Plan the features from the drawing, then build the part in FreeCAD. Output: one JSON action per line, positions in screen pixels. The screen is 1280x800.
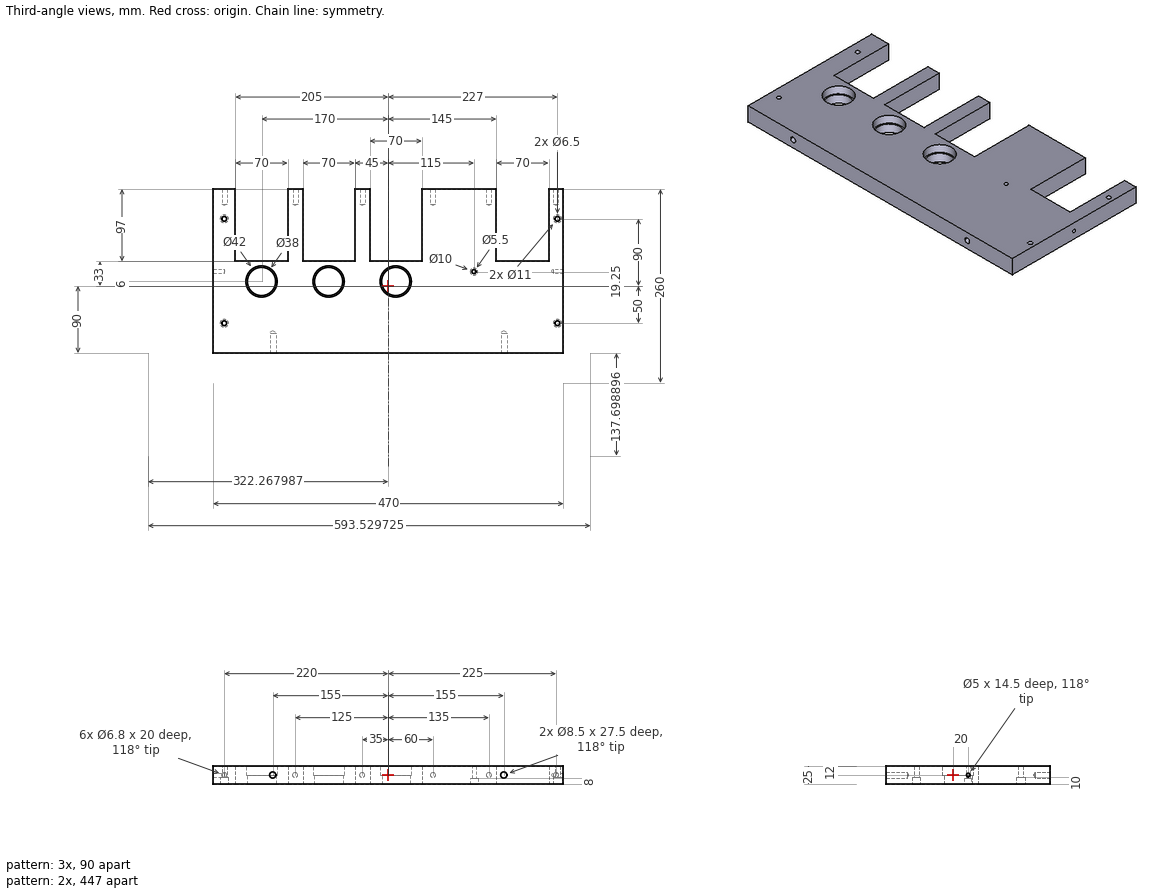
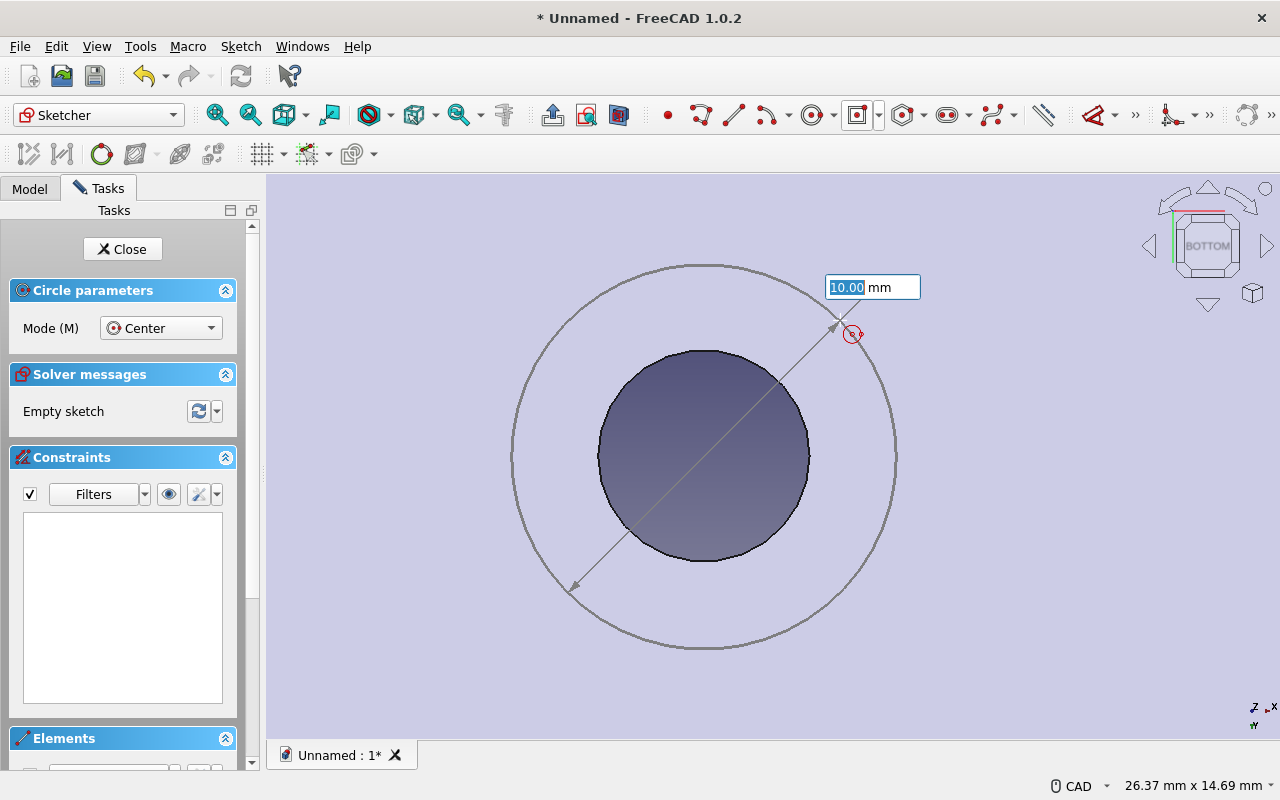
{"action": "type", "text": "10"}
{"action": "key", "text": "Return"}
{"action": "key", "text": "Escape"}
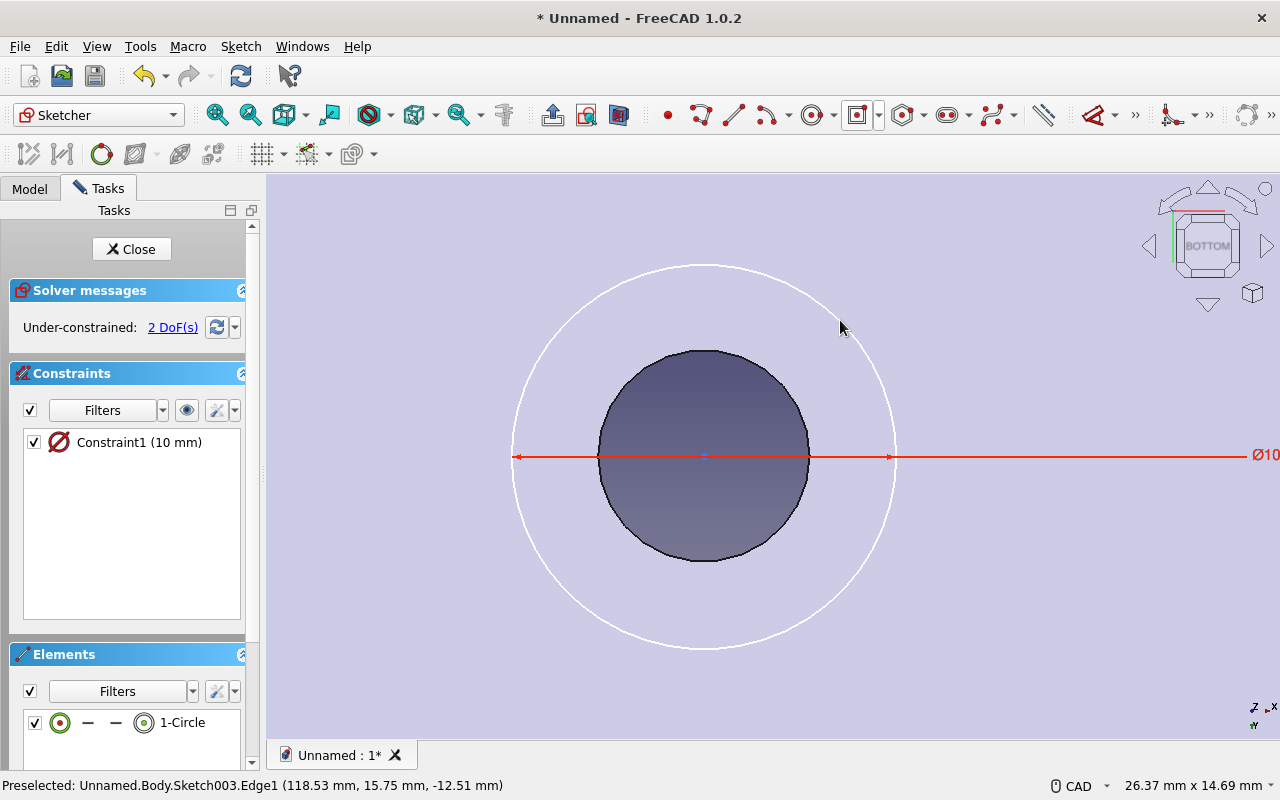
{"action": "left_click", "coordinate": [1092, 116]}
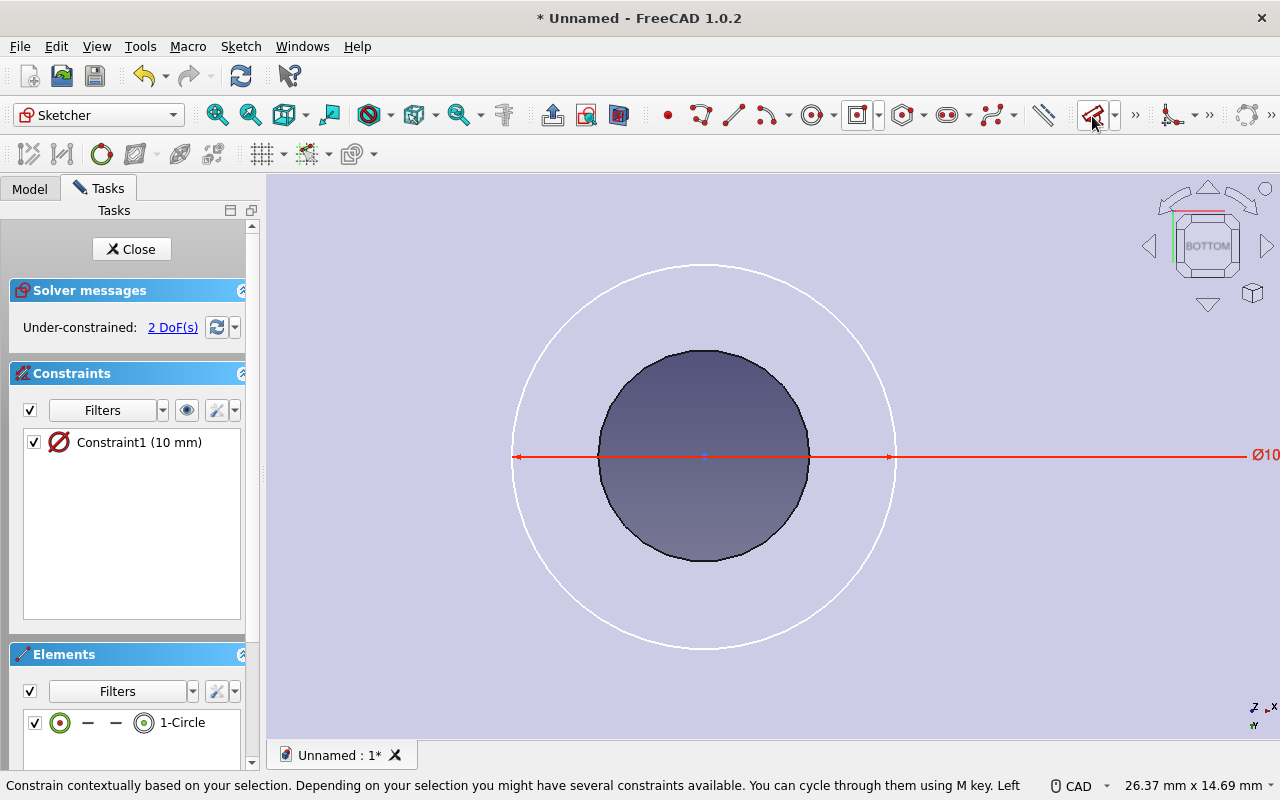
{"action": "left_click", "coordinate": [704, 457]}
{"action": "left_click", "coordinate": [499, 491]}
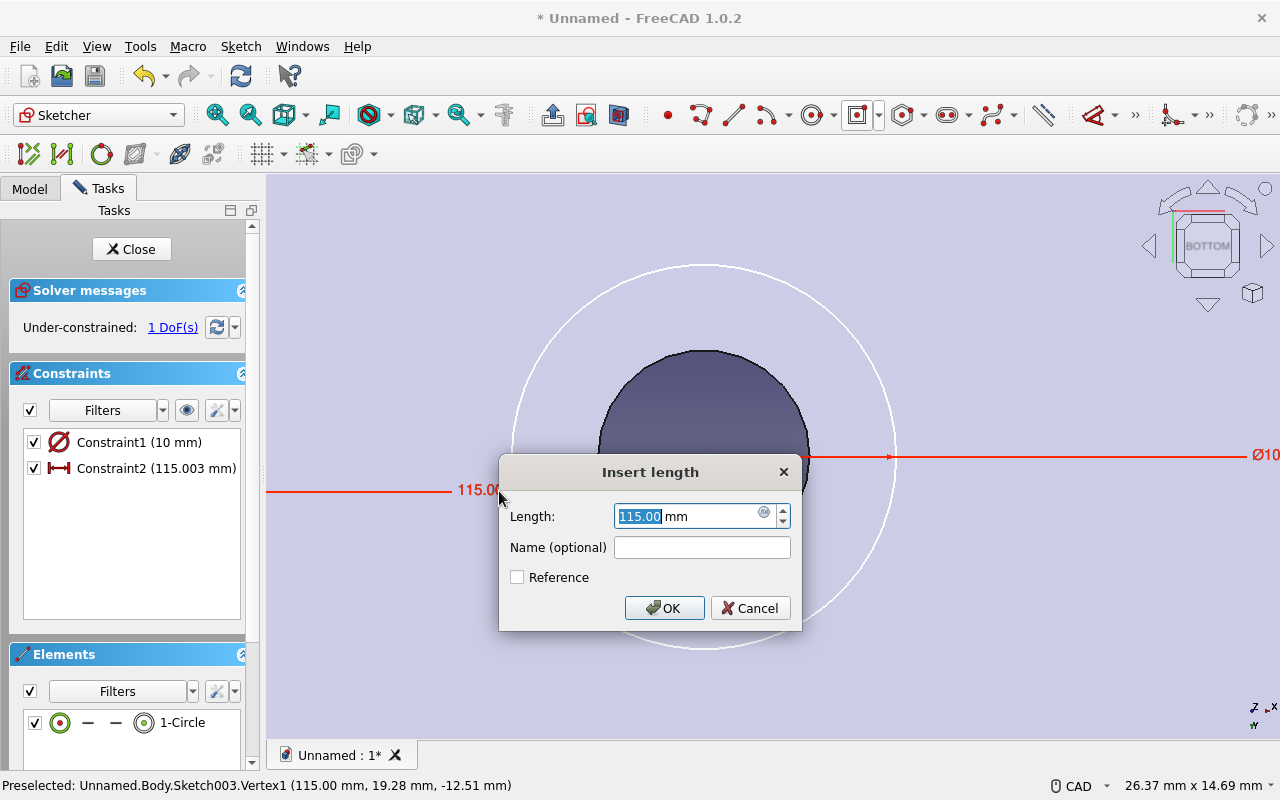
{"action": "type", "text": "115"}
{"action": "key", "text": "Return"}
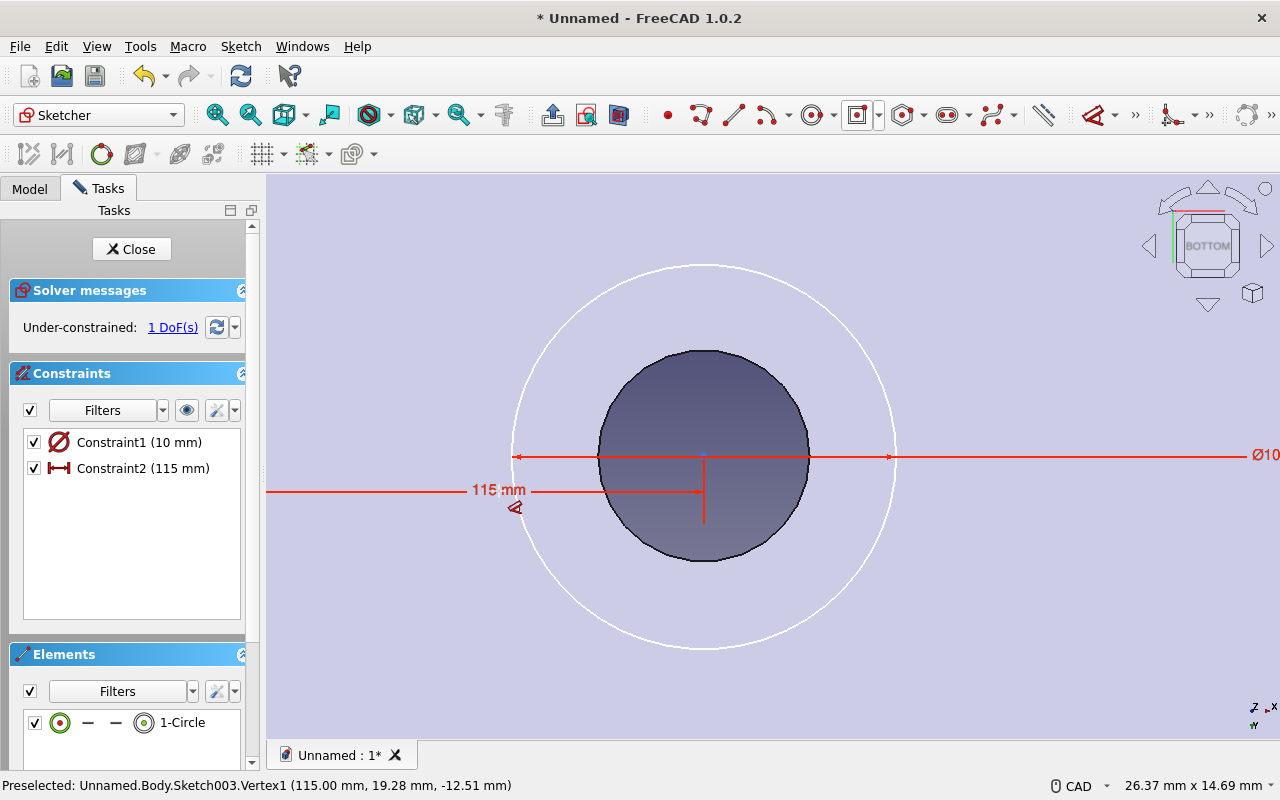
{"action": "left_click", "coordinate": [704, 457]}
{"action": "left_click", "coordinate": [738, 330]}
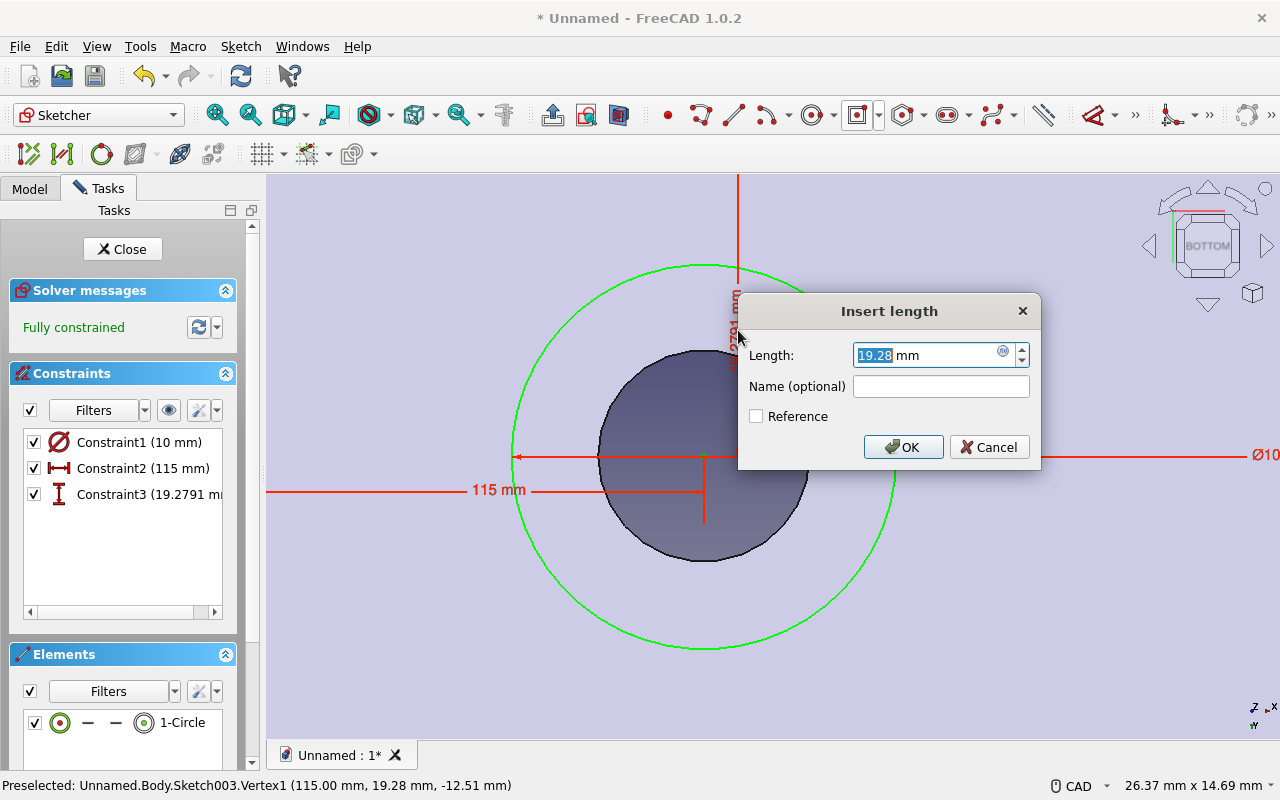
{"action": "type", "text": "19.25"}
{"action": "key", "text": "Return"}
{"action": "key", "text": "Escape"}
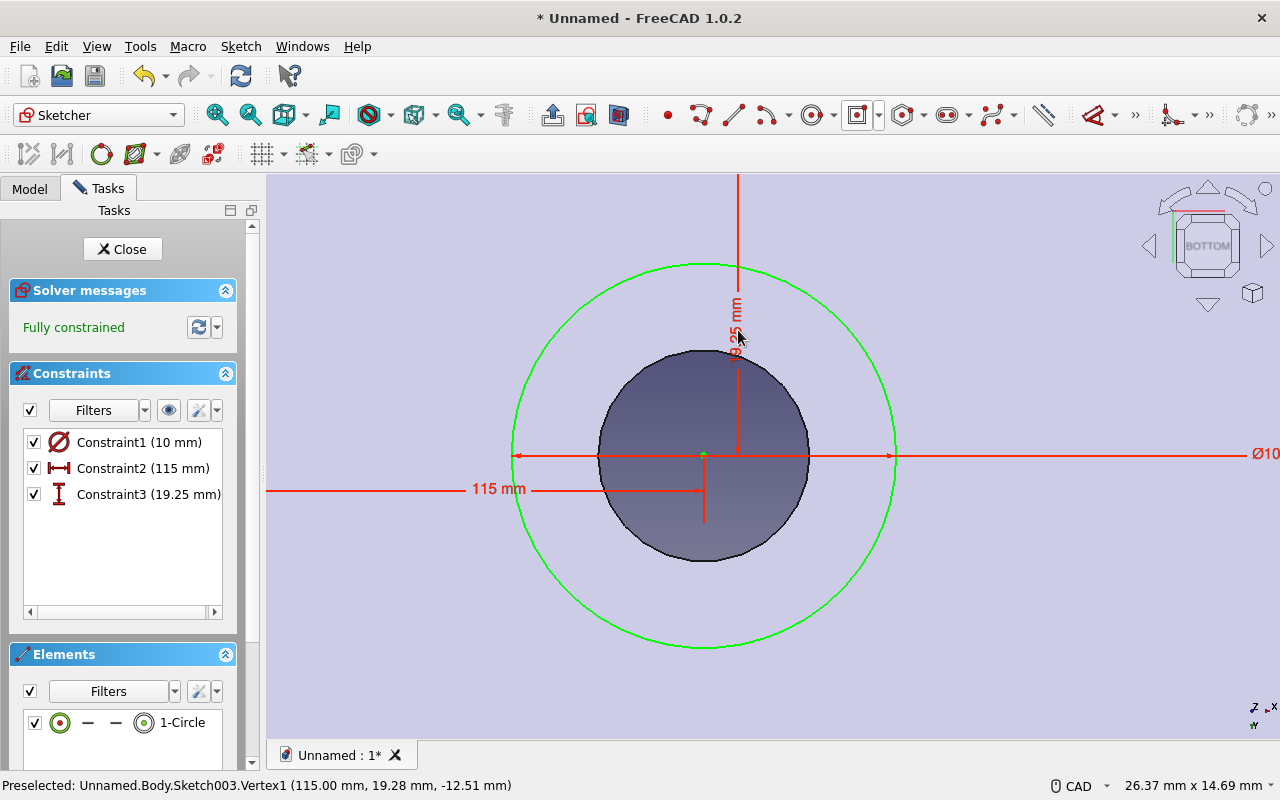
{"action": "left_click", "coordinate": [123, 249]}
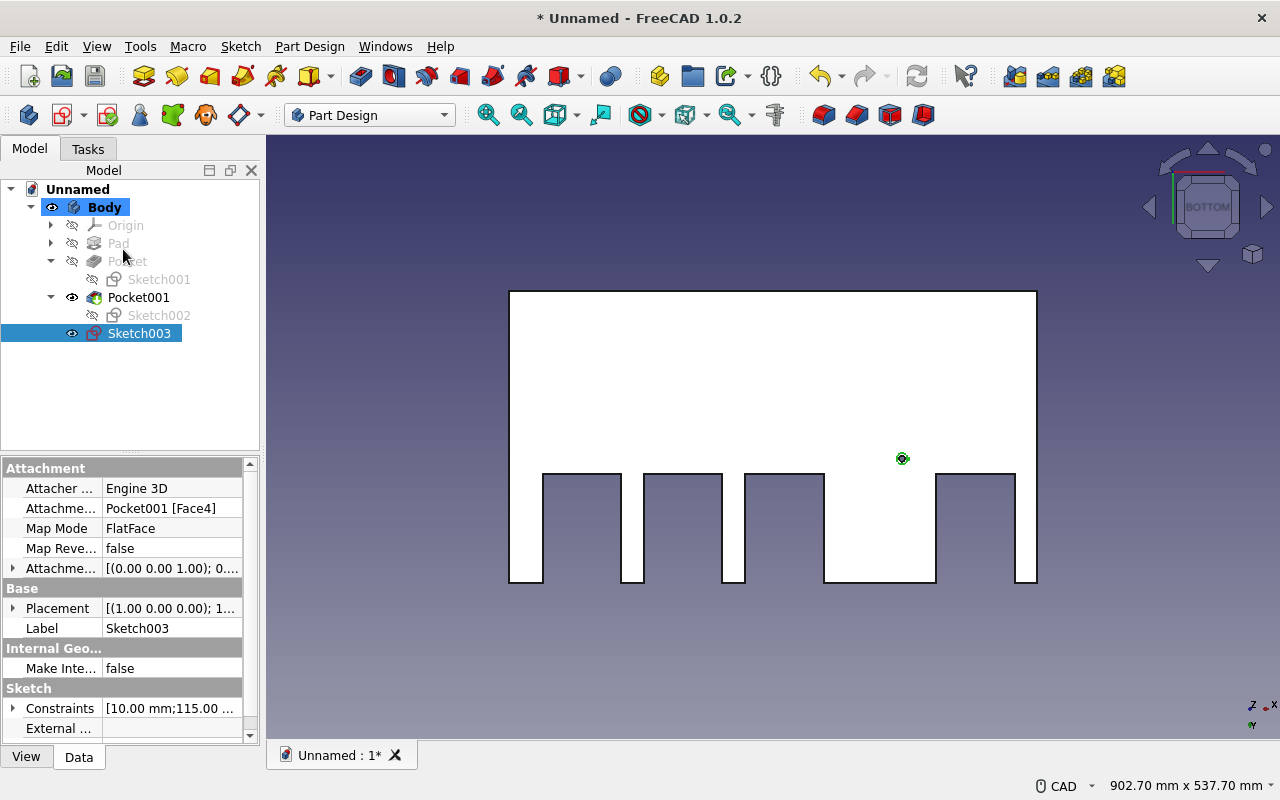
{"action": "left_click", "coordinate": [361, 76]}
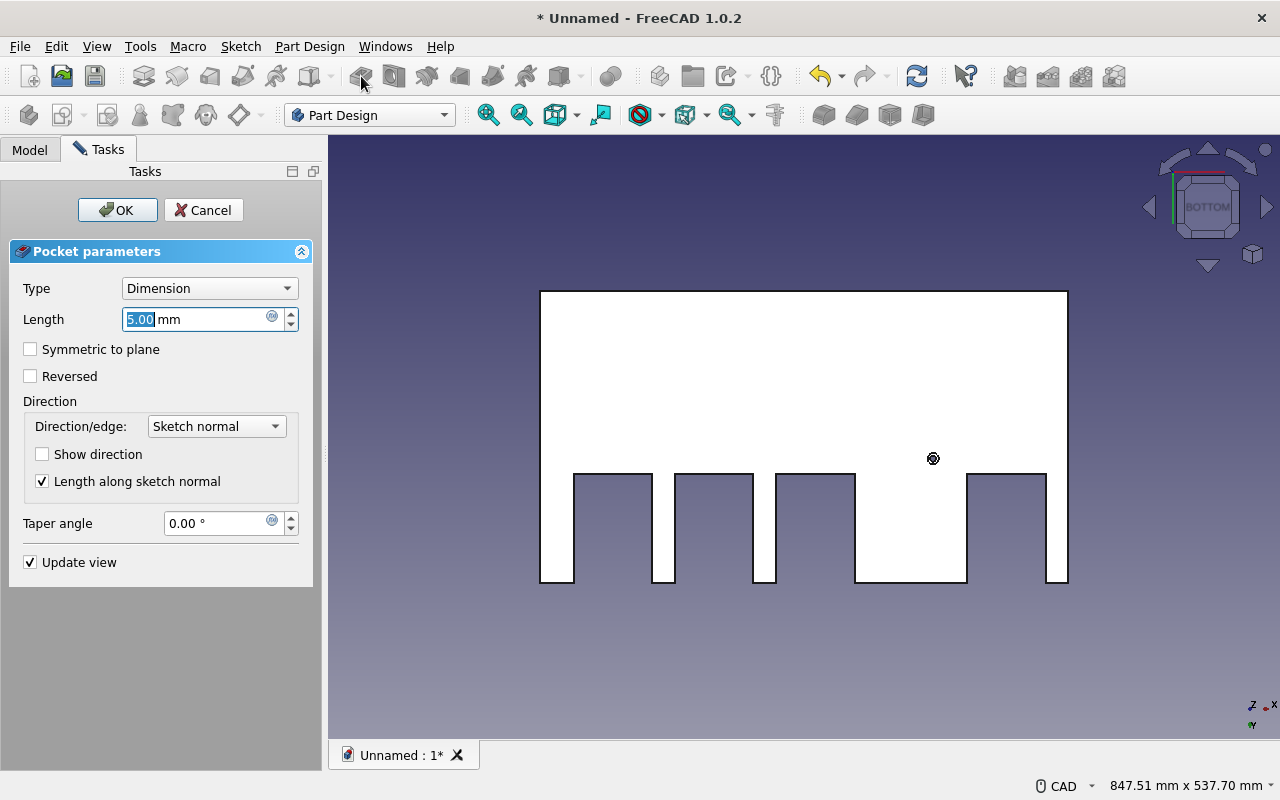
{"action": "type", "text": "8"}
{"action": "key", "text": "Tab"}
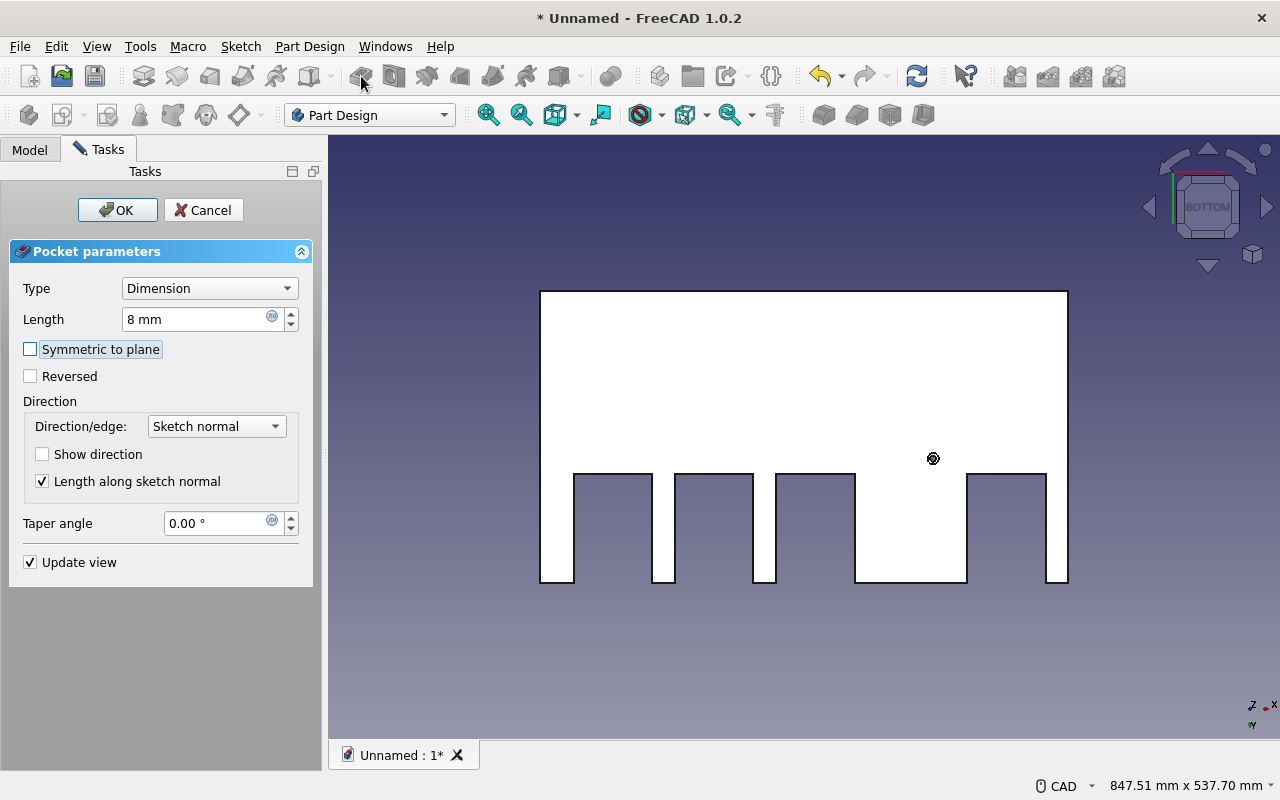
{"action": "left_click", "coordinate": [118, 210]}